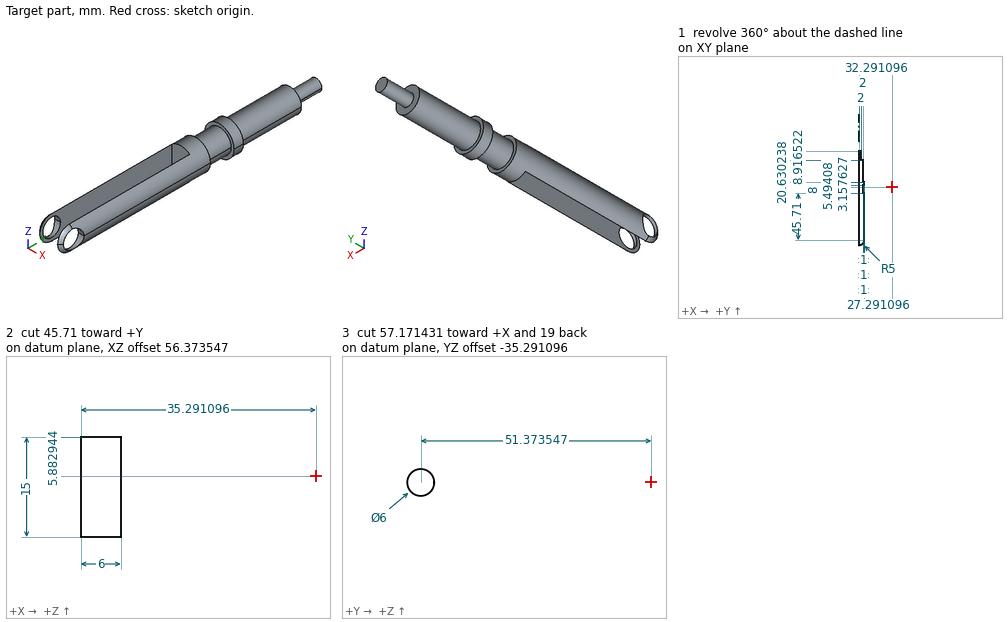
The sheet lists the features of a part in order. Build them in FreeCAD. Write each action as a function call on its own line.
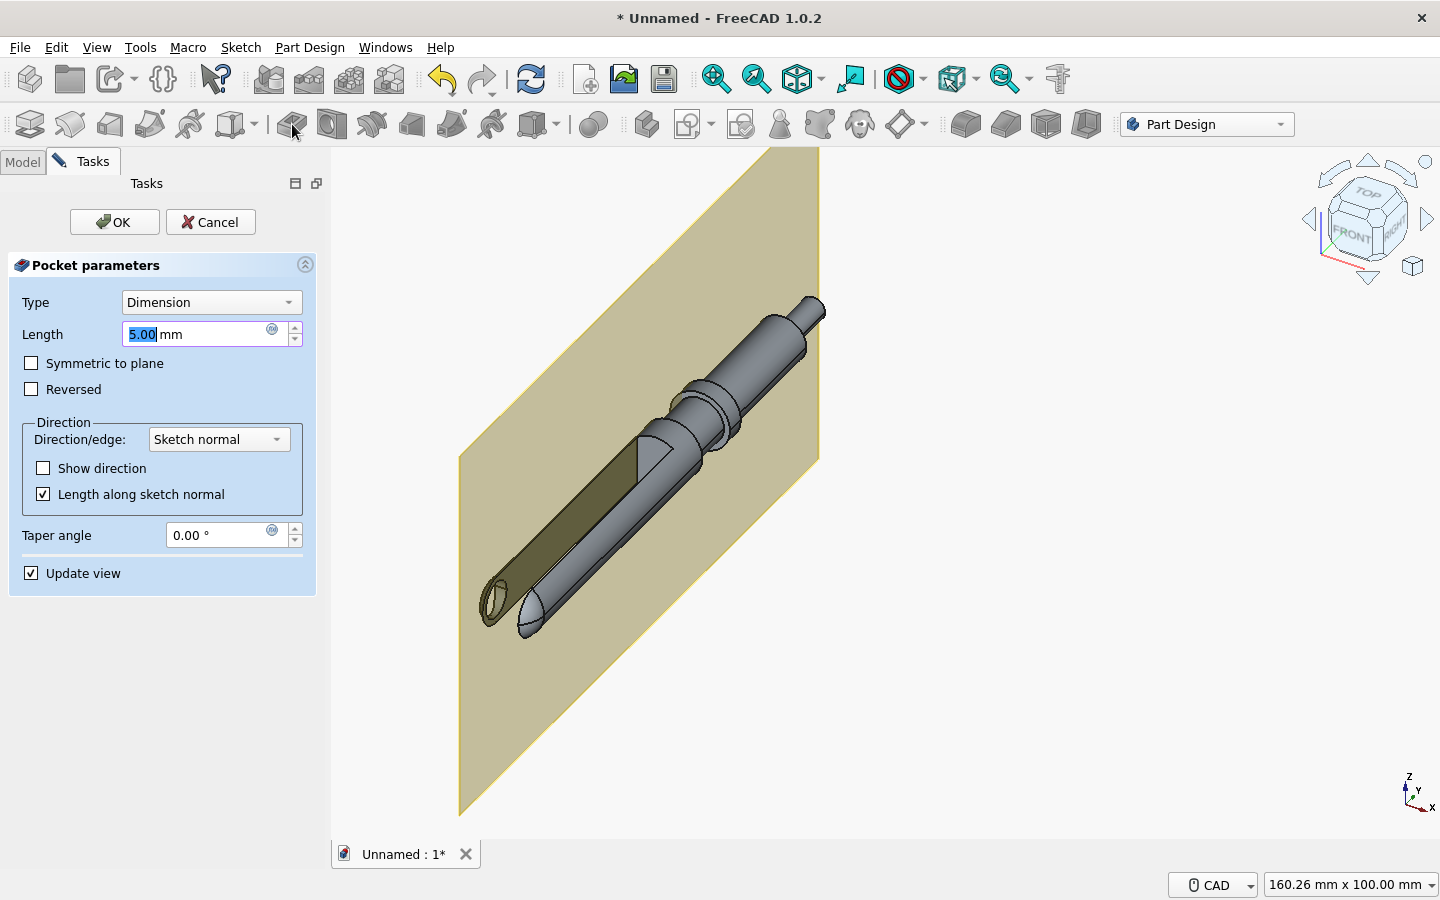
click(212, 302)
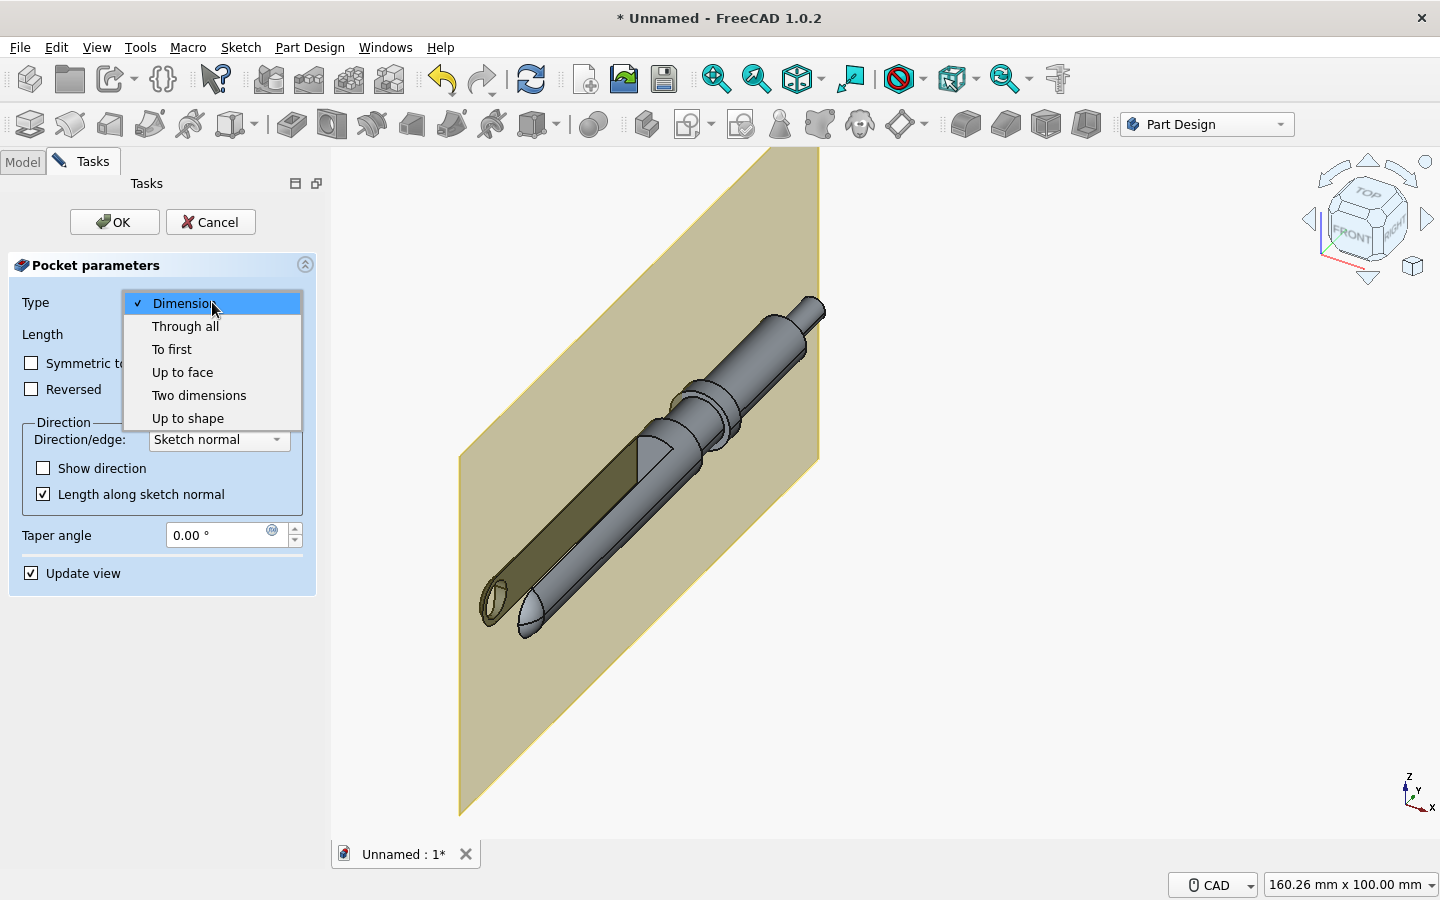
click(212, 396)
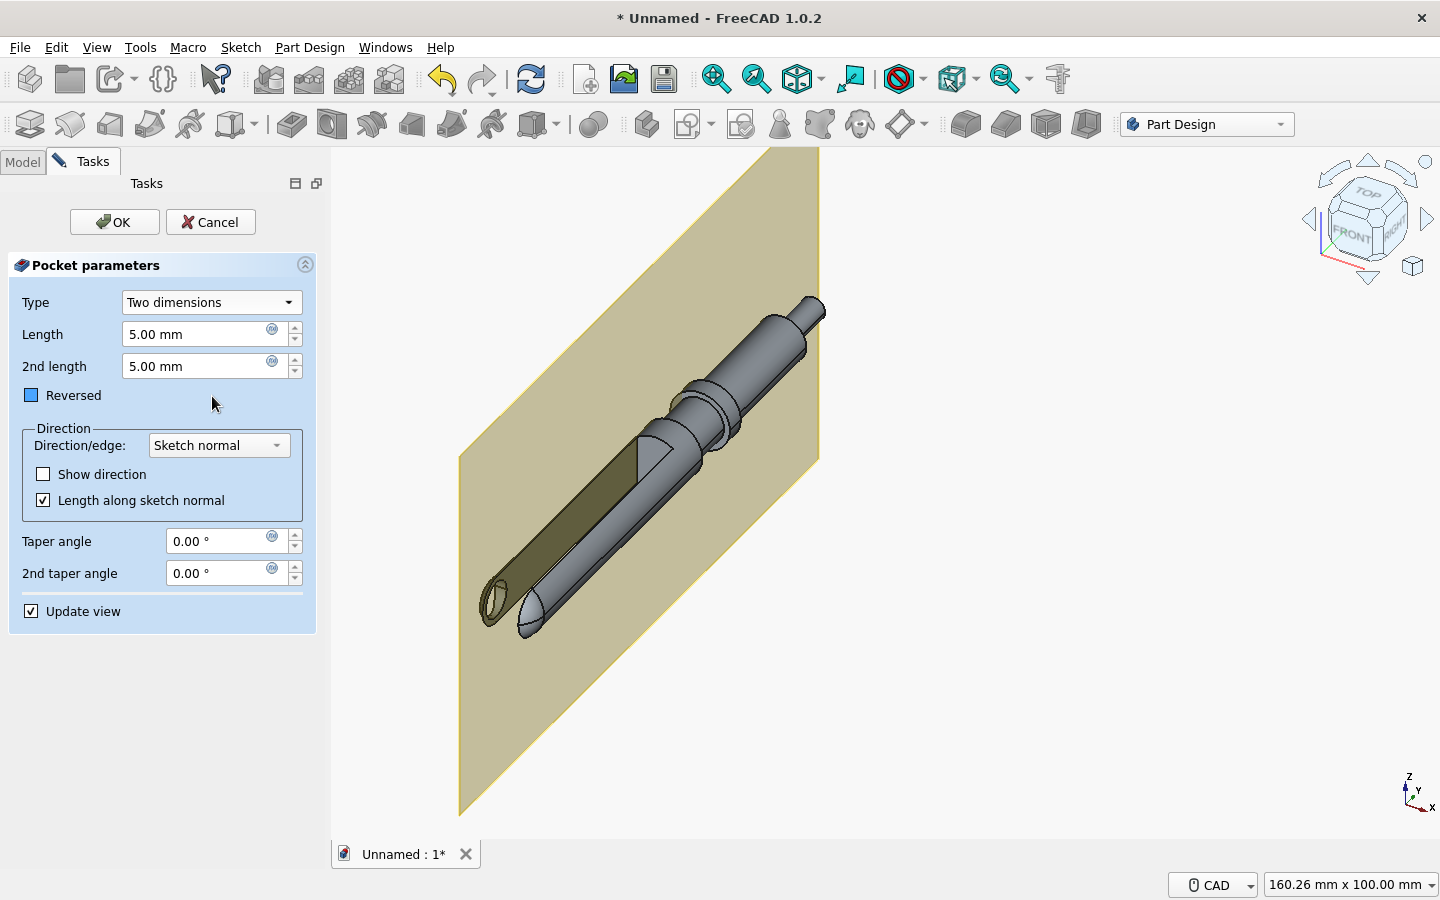
triple_click(204, 334)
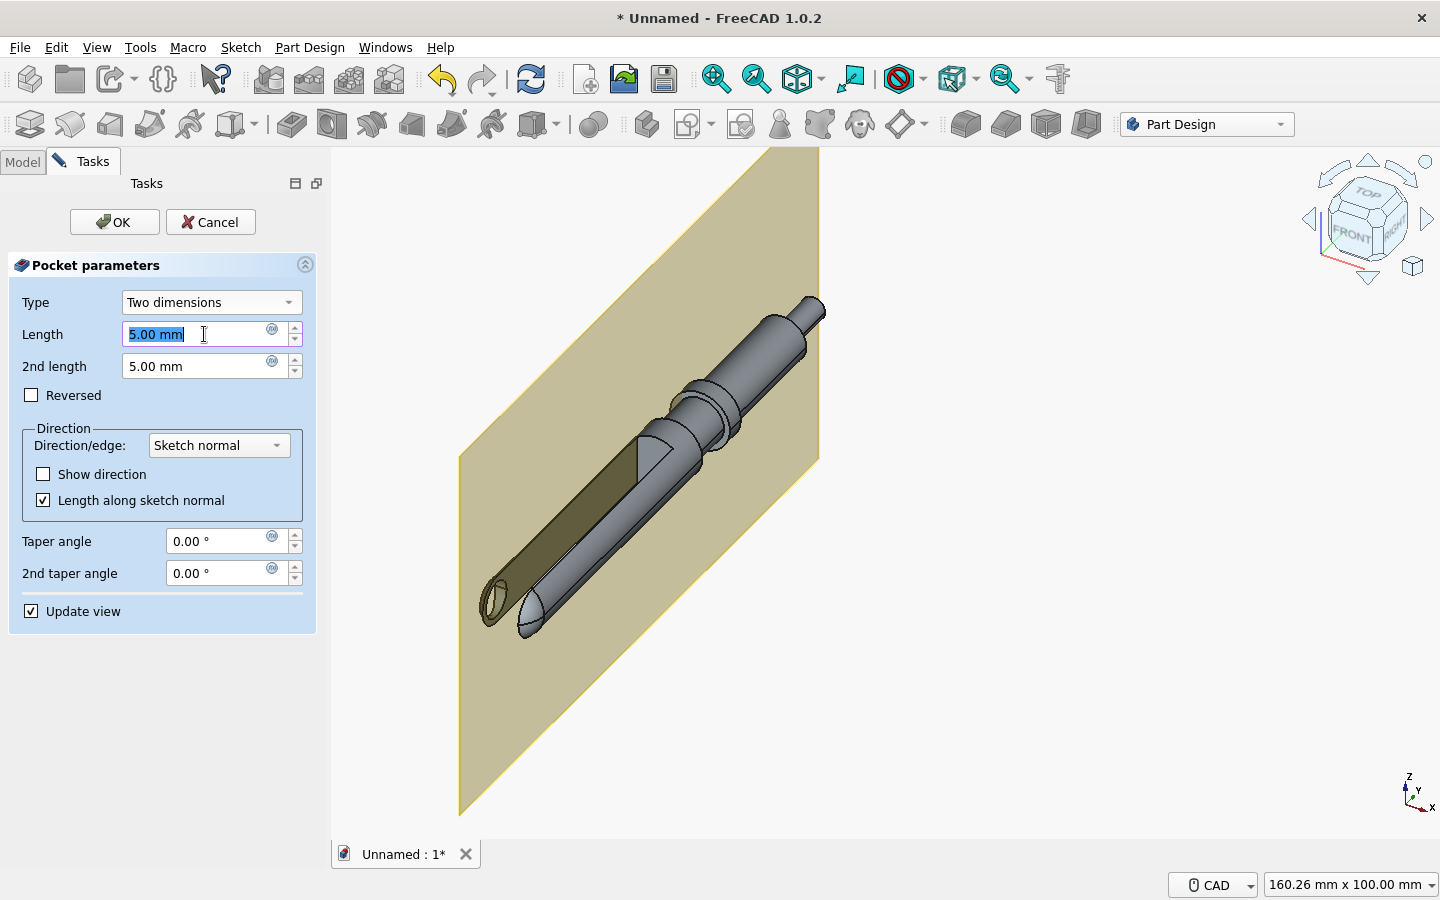
text(57.171431)
key(Tab)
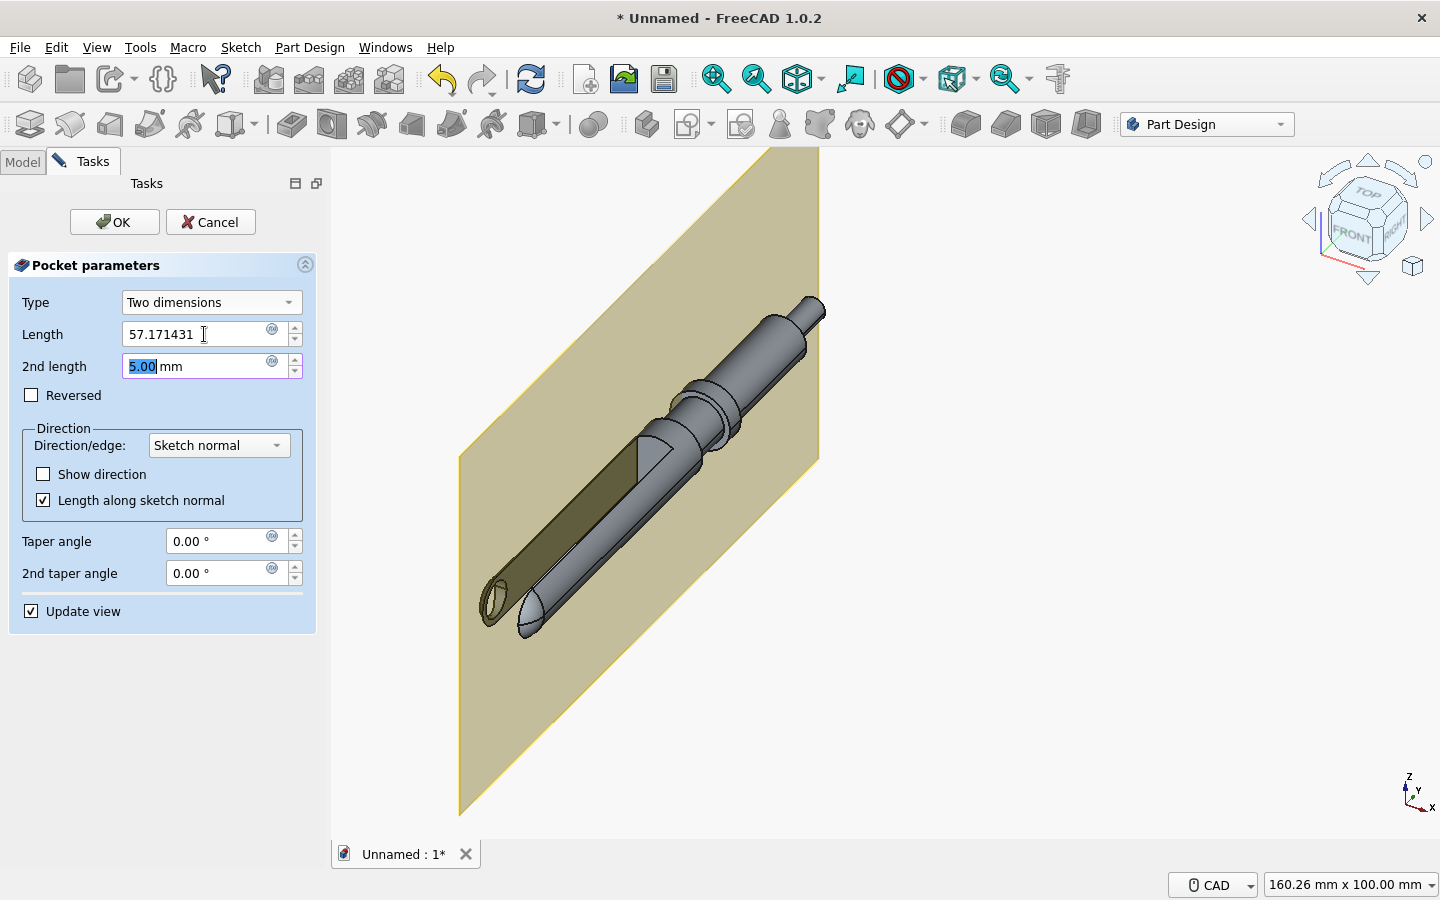
text(19)
key(Tab)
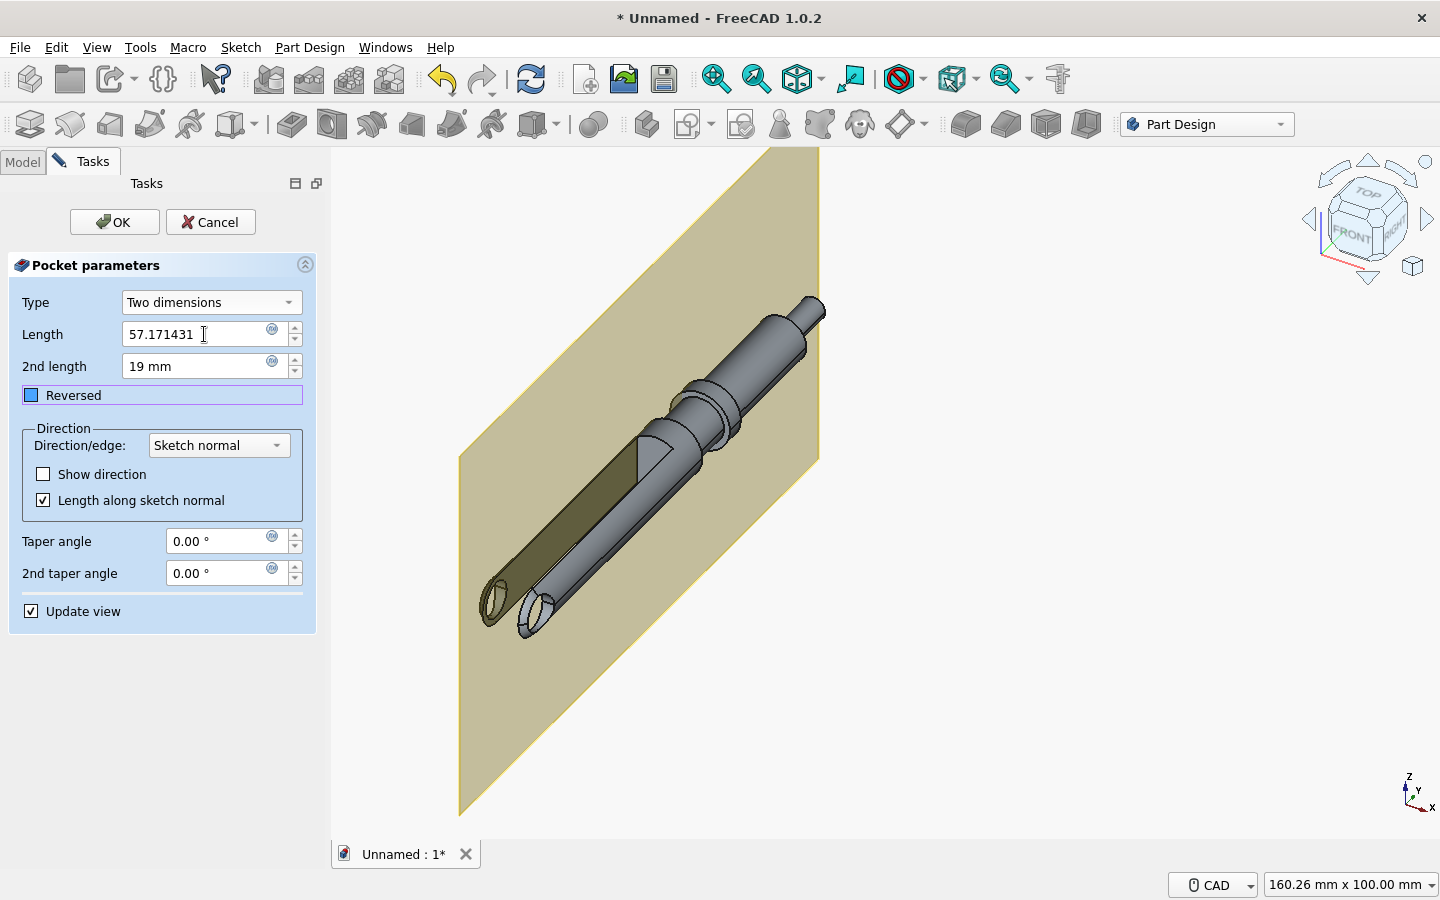
click(30, 395)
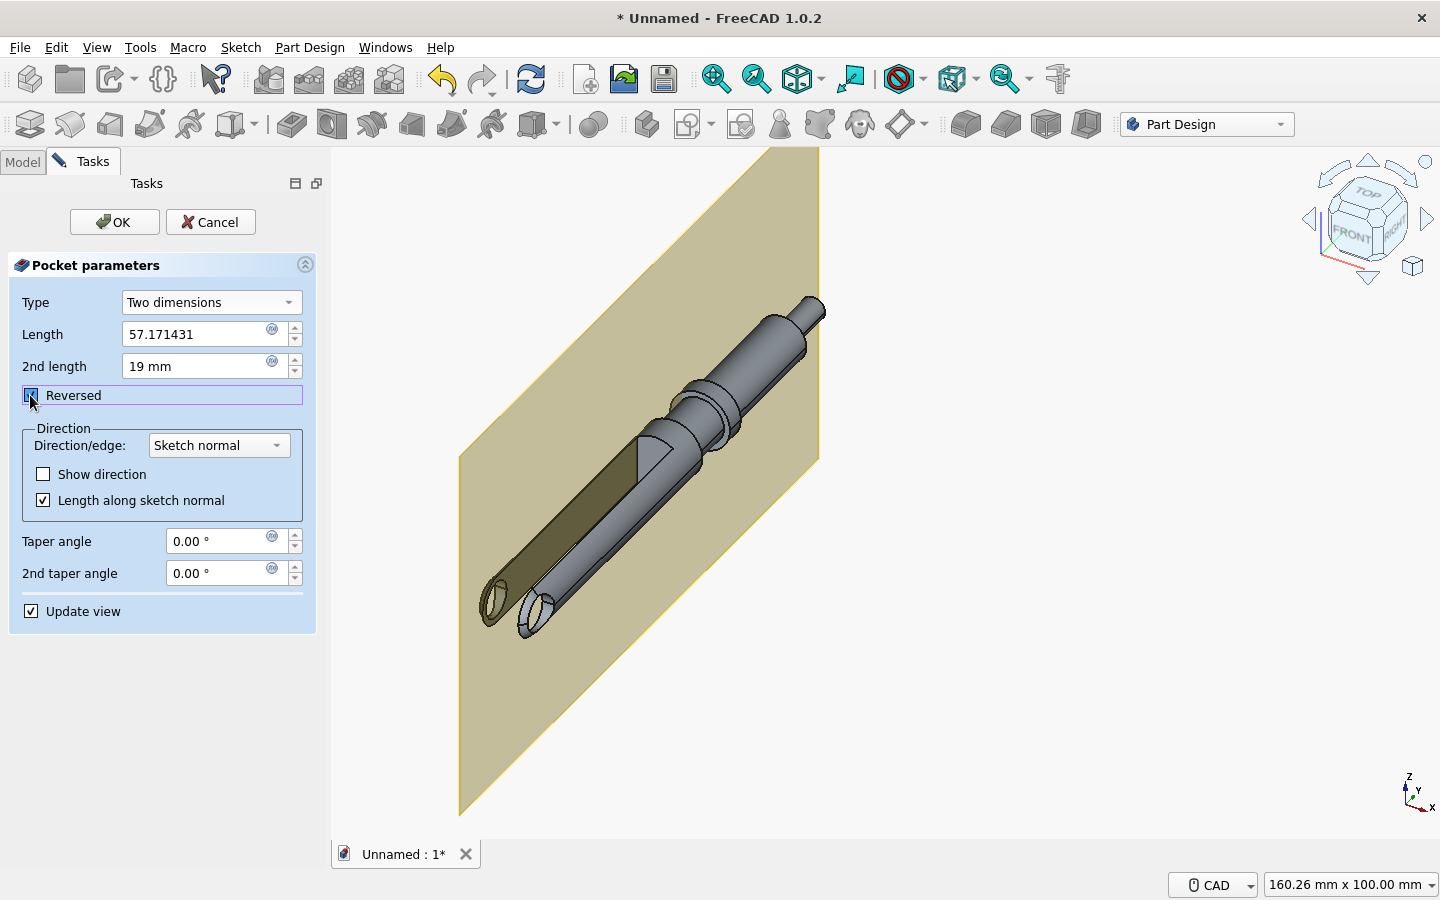
click(115, 222)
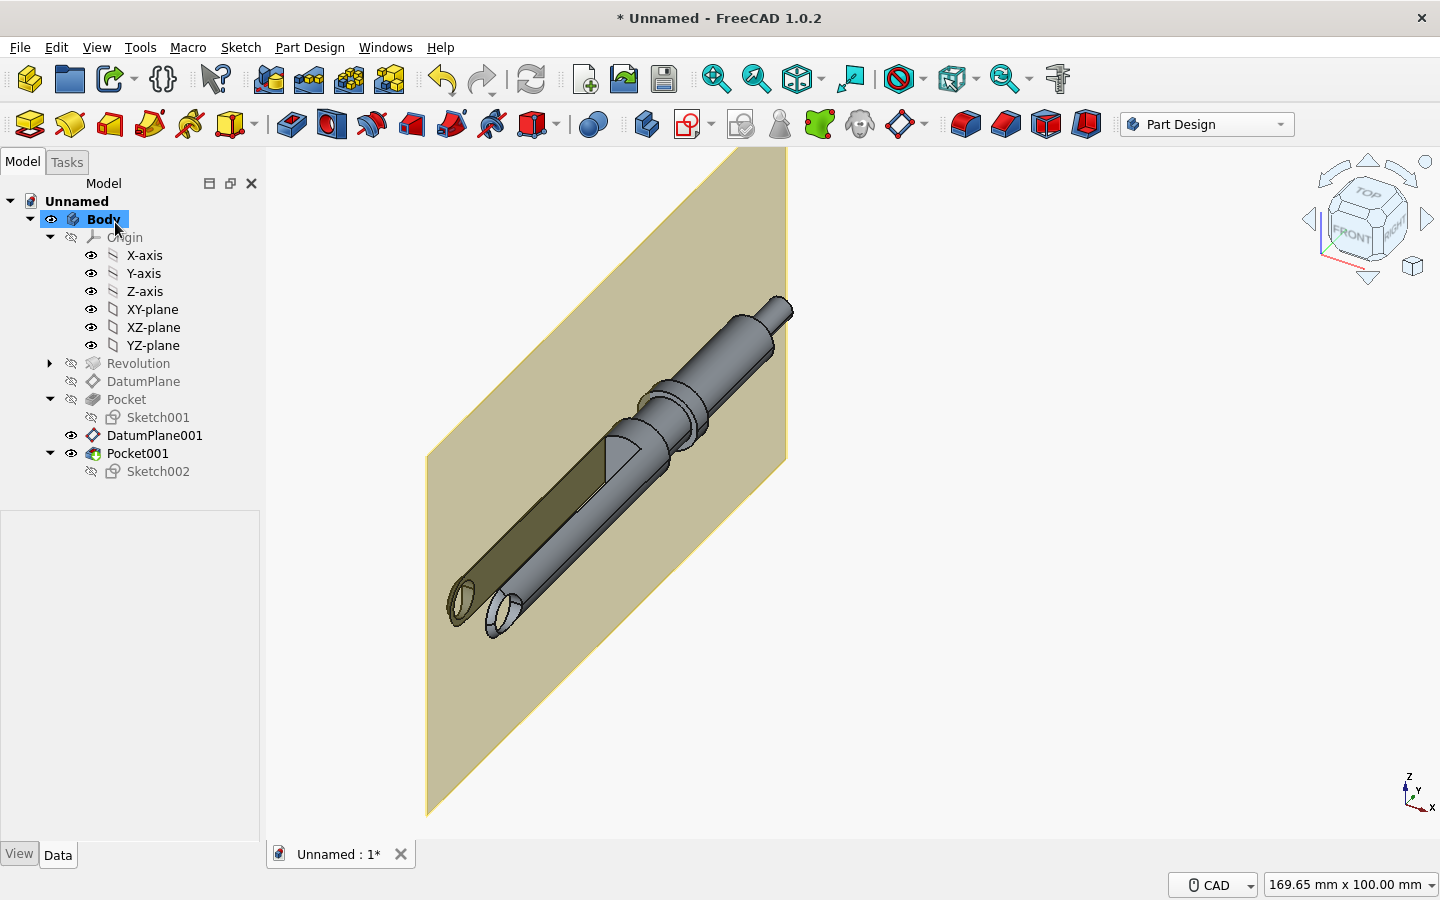
click(116, 435)
key(space)